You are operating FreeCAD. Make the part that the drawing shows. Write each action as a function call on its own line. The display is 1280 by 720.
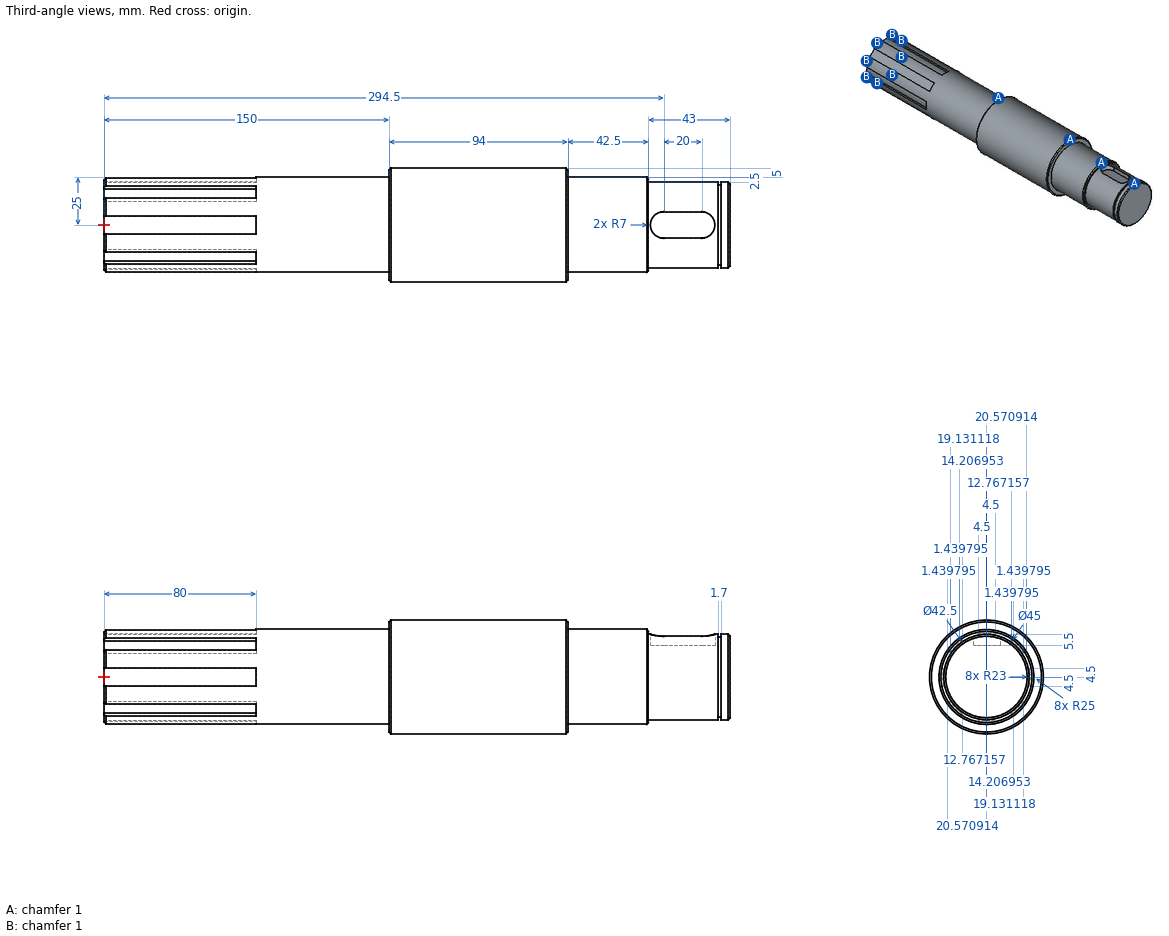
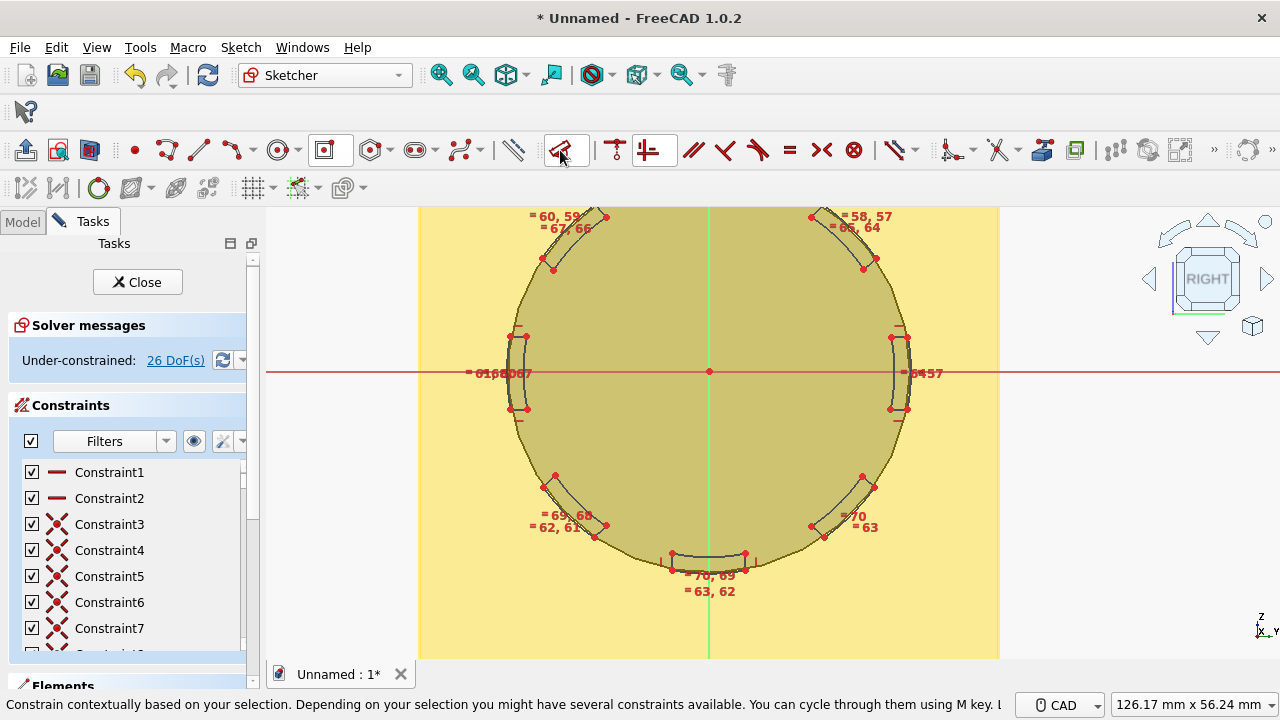
click(894, 388)
click(926, 391)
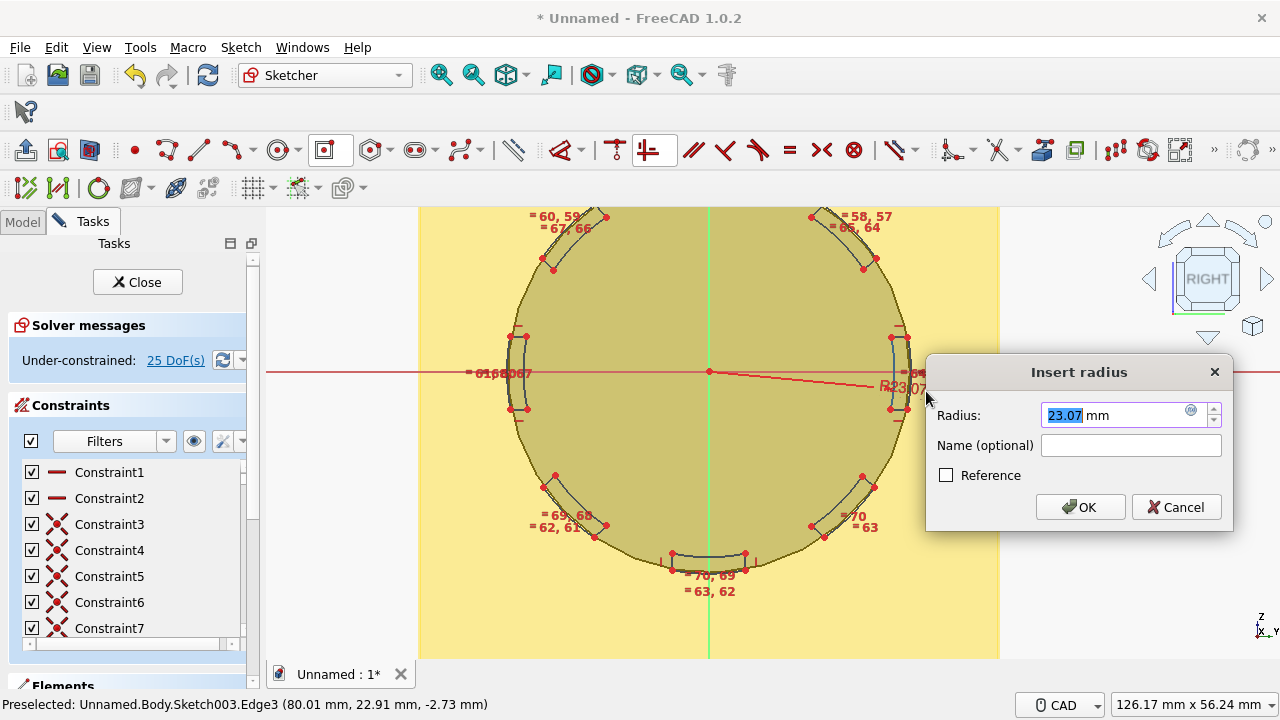
text(23)
key(Return)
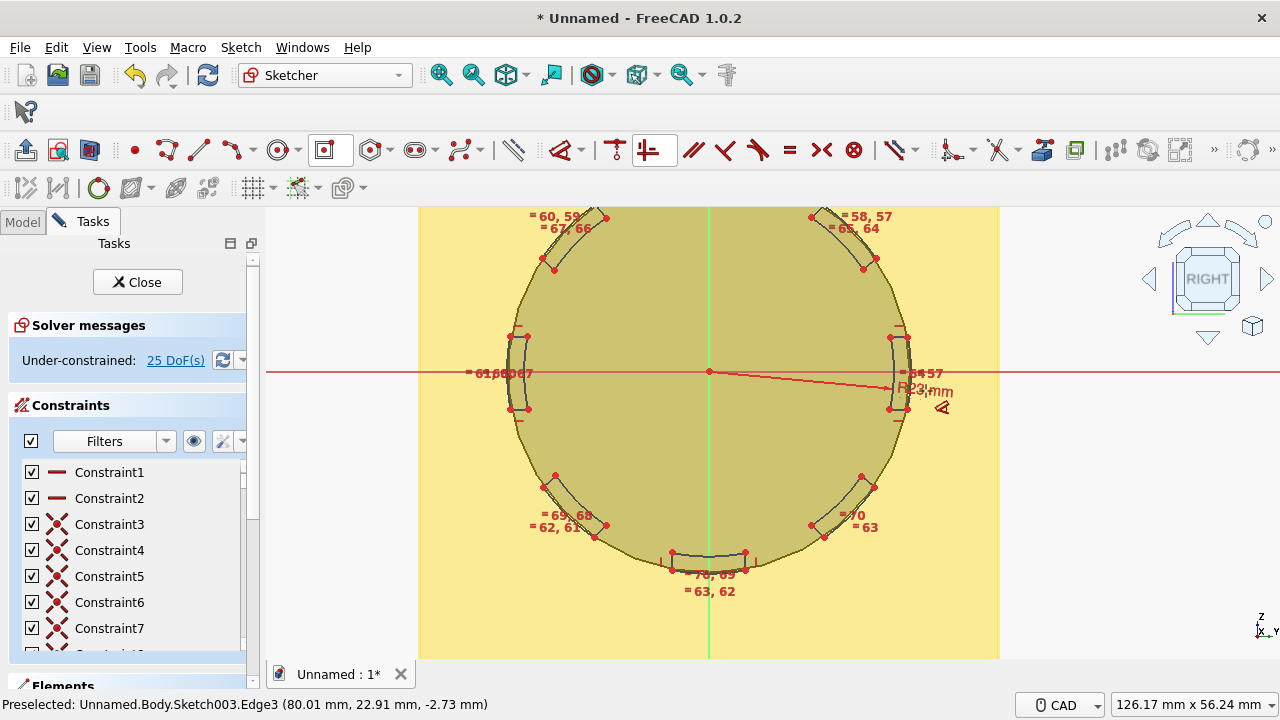
click(910, 388)
click(904, 500)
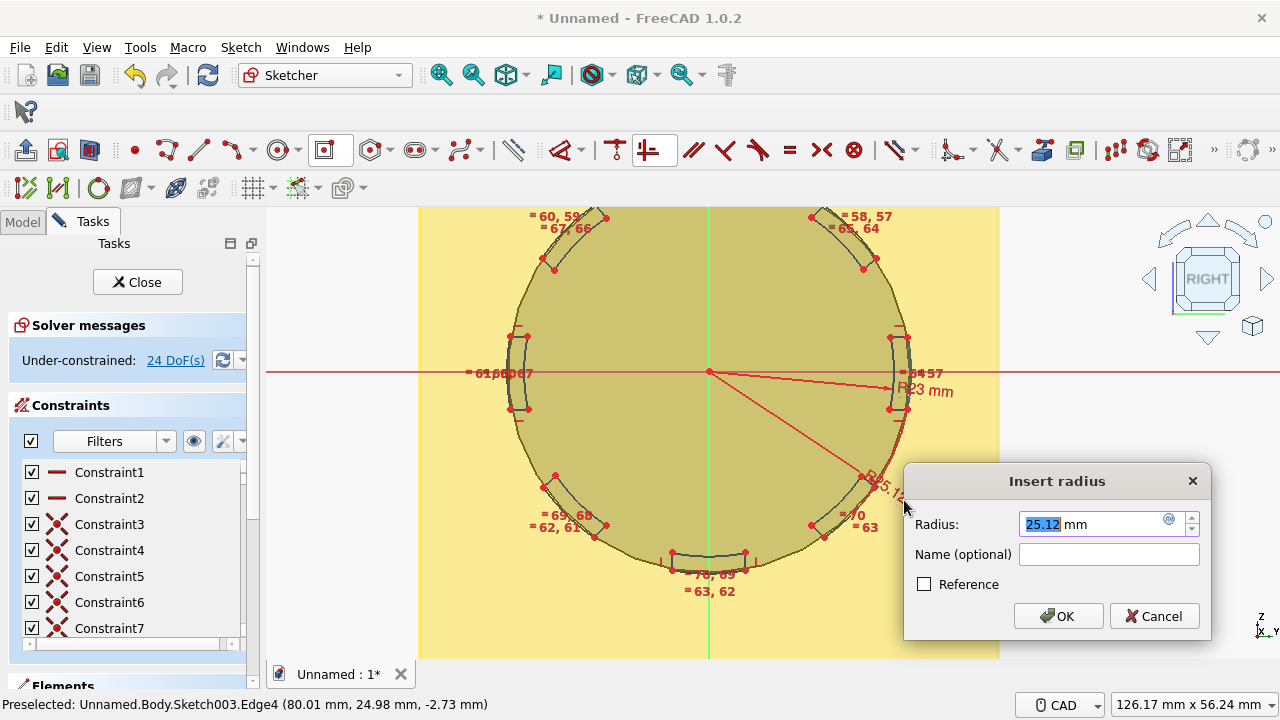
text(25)
key(Return)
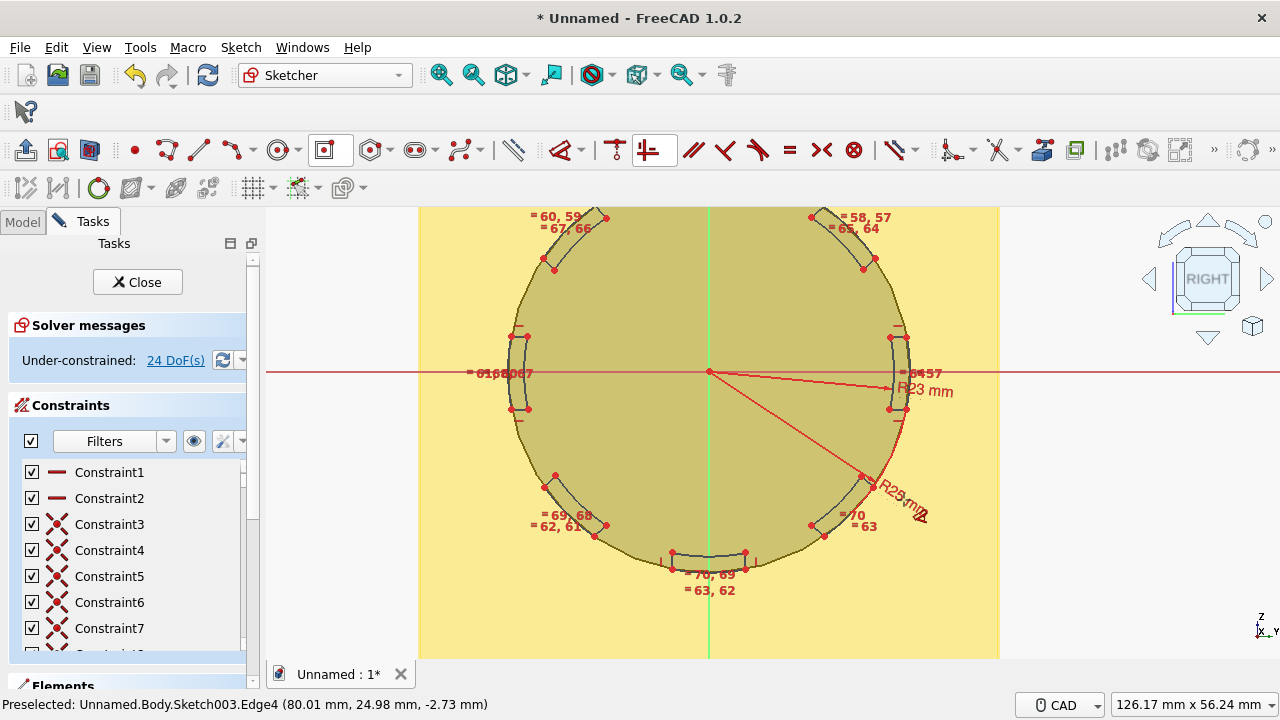
click(906, 410)
click(675, 391)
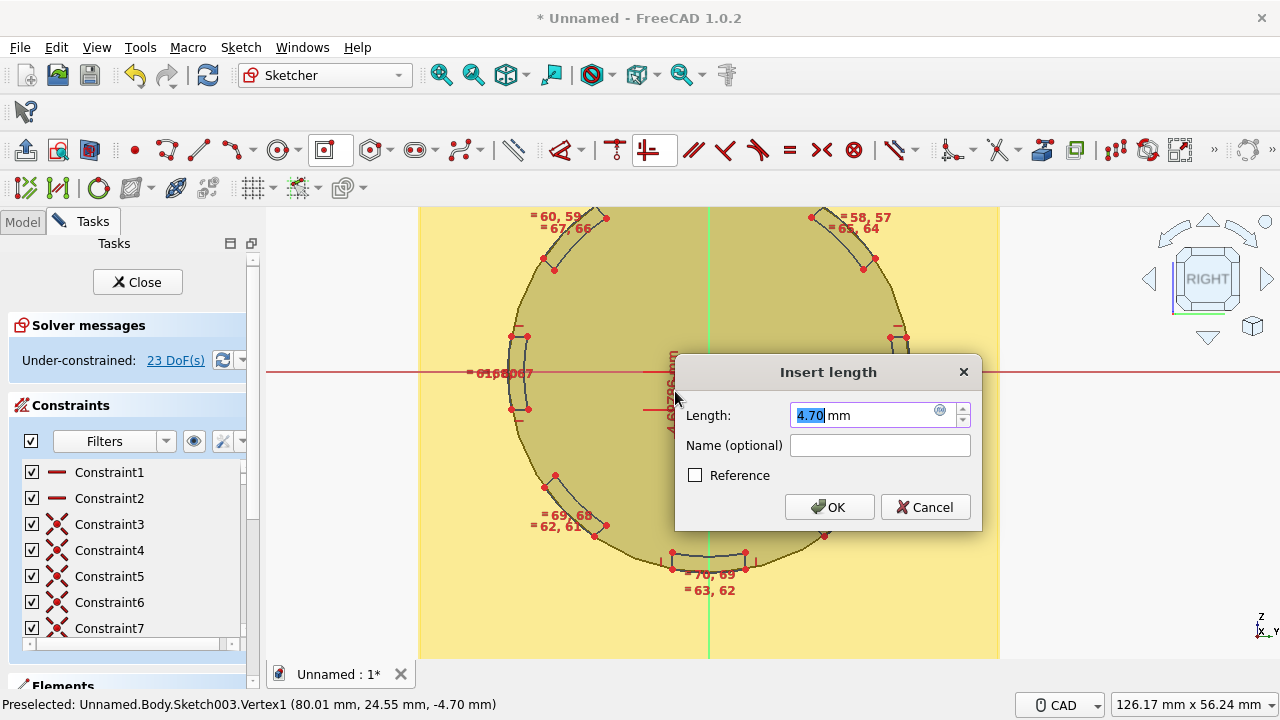
text(4.5)
key(Return)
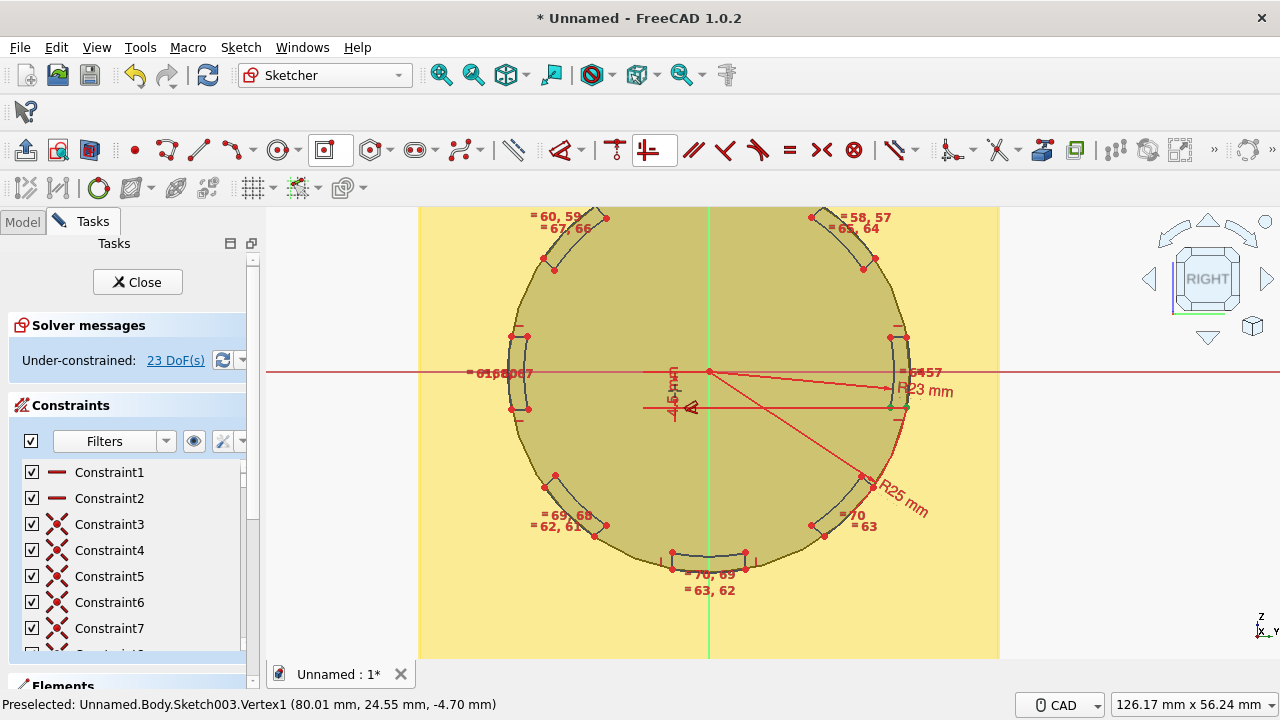
click(891, 337)
click(925, 354)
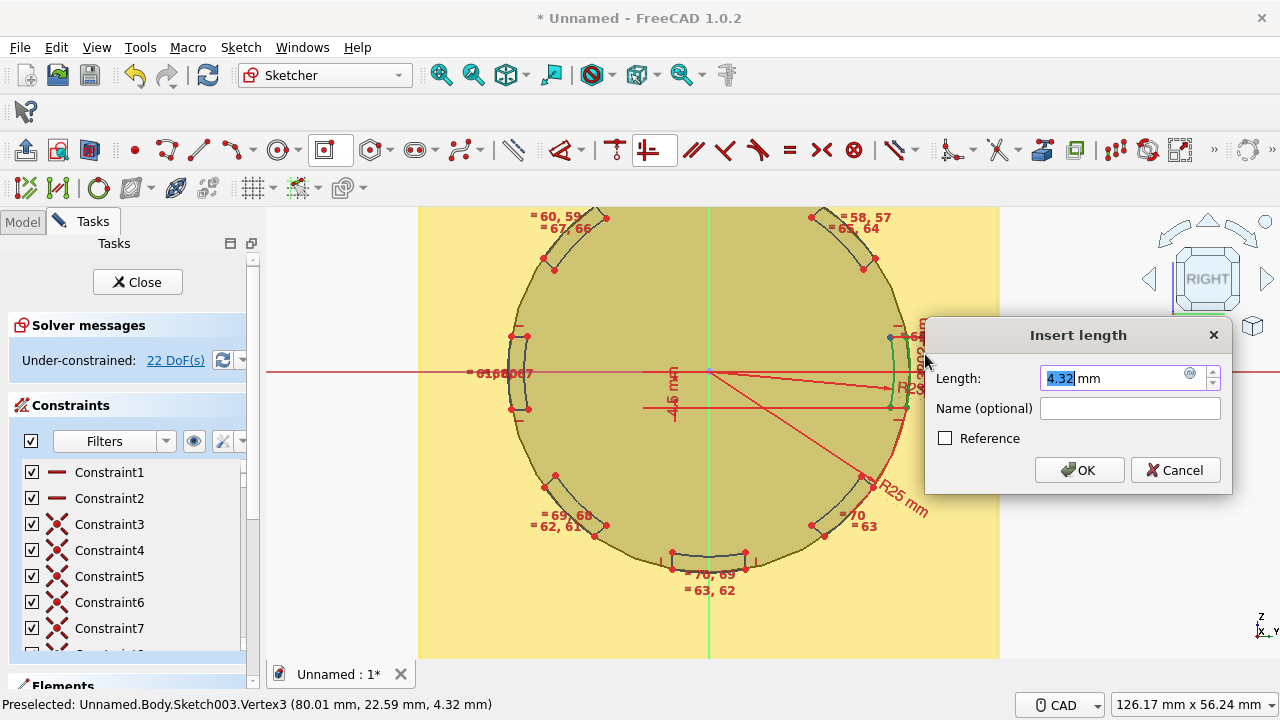
text(4.5)
key(Return)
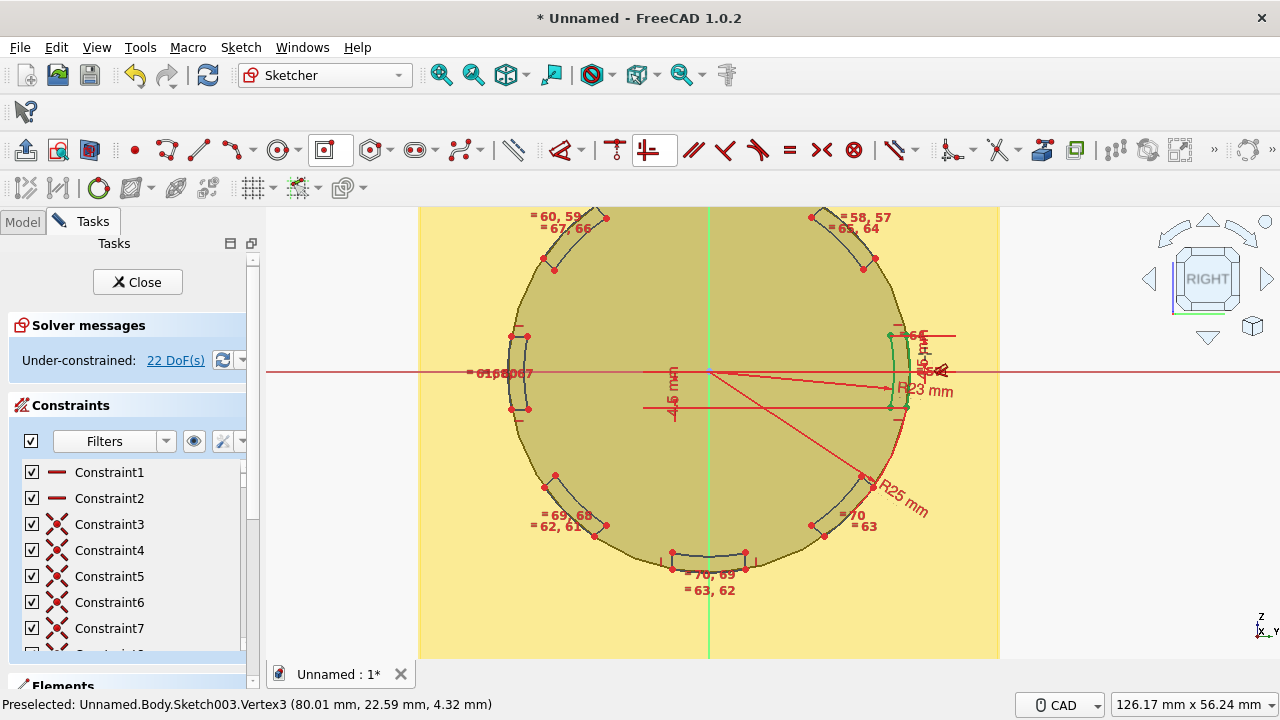
scroll(695, 558, down, 2)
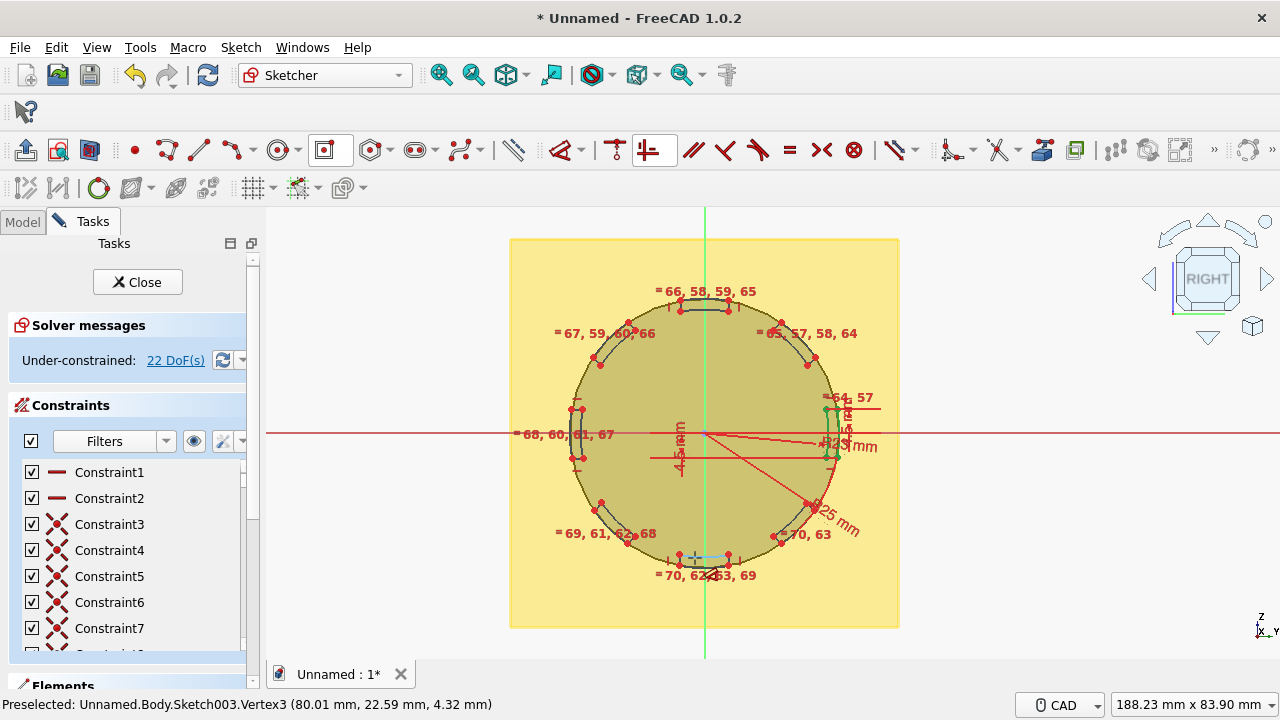
scroll(681, 312, up, 3)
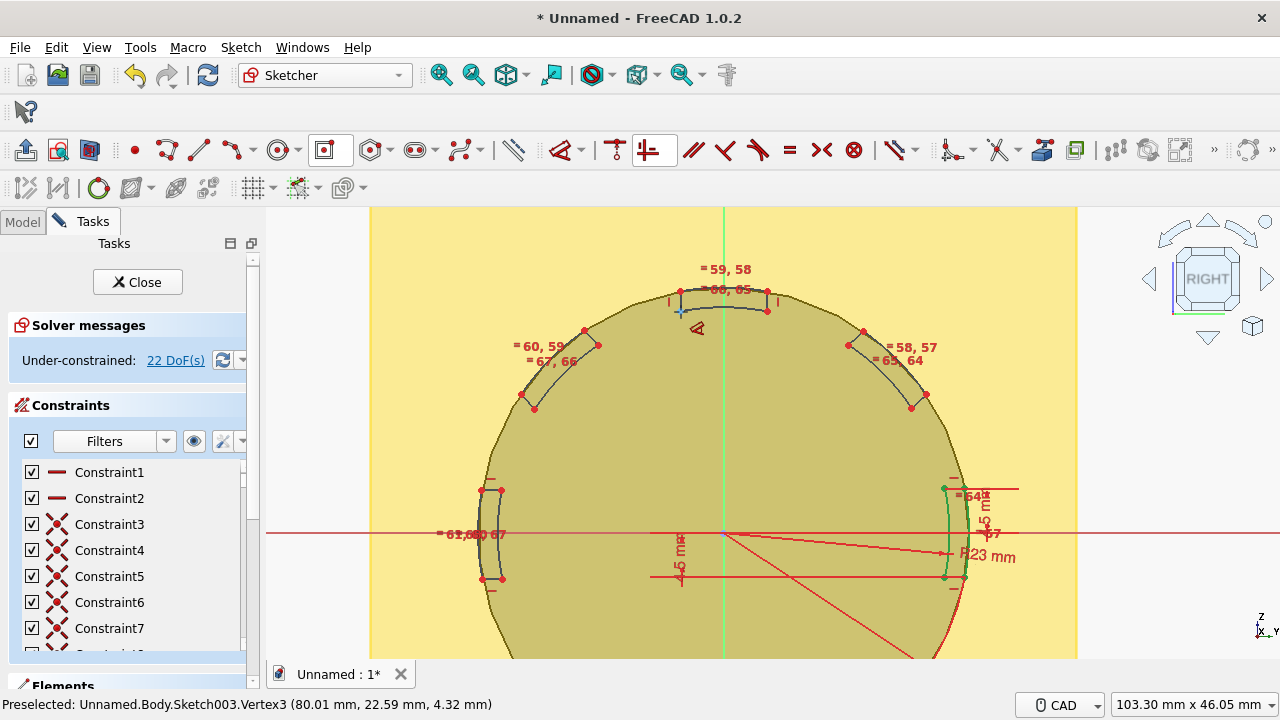
click(681, 311)
click(702, 253)